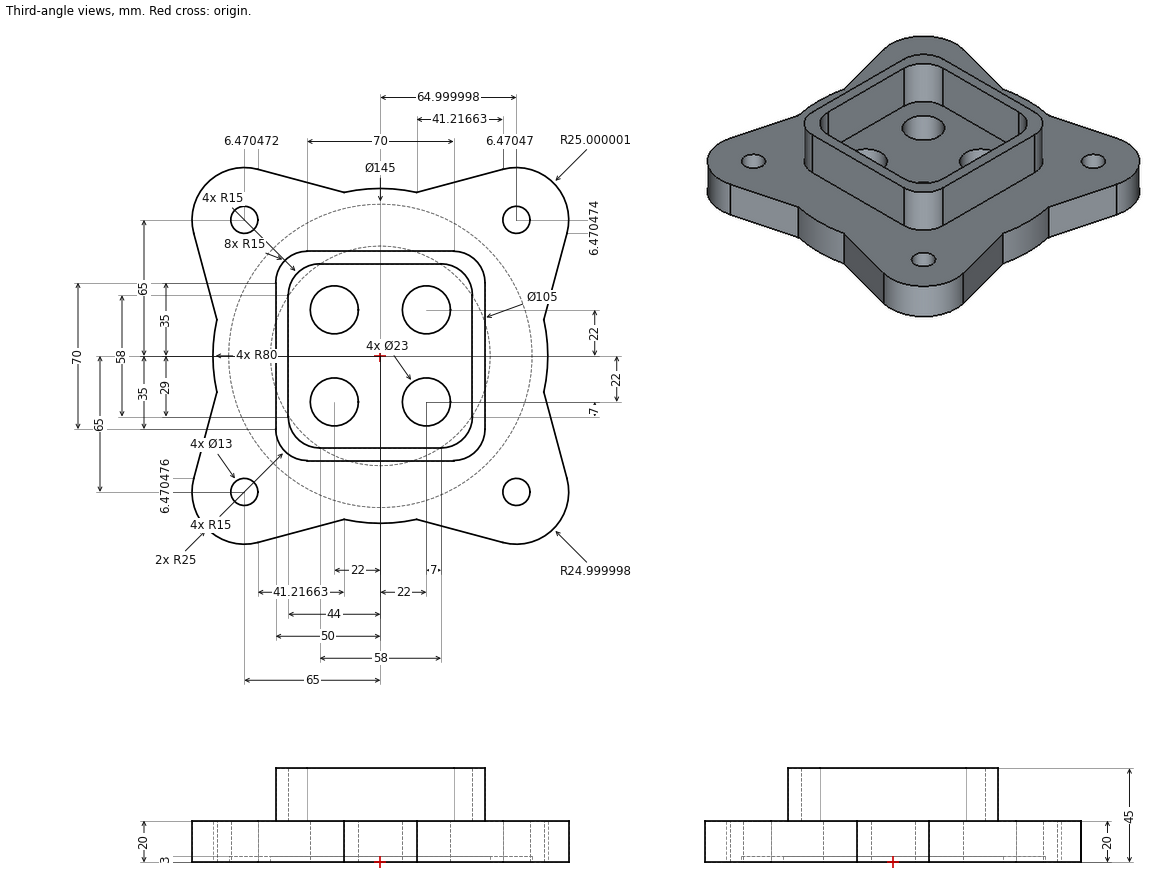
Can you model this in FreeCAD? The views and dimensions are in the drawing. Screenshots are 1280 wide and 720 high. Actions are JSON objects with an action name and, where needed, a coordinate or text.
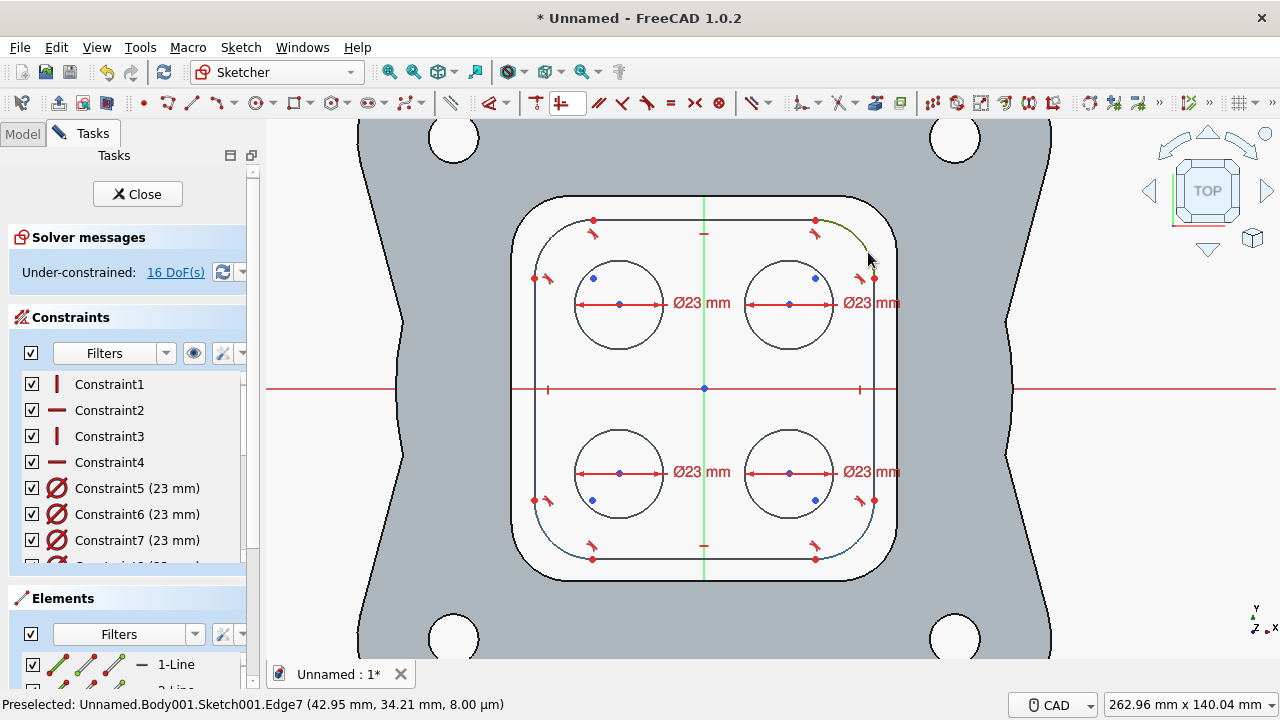
{"action": "left_click", "coordinate": [567, 226]}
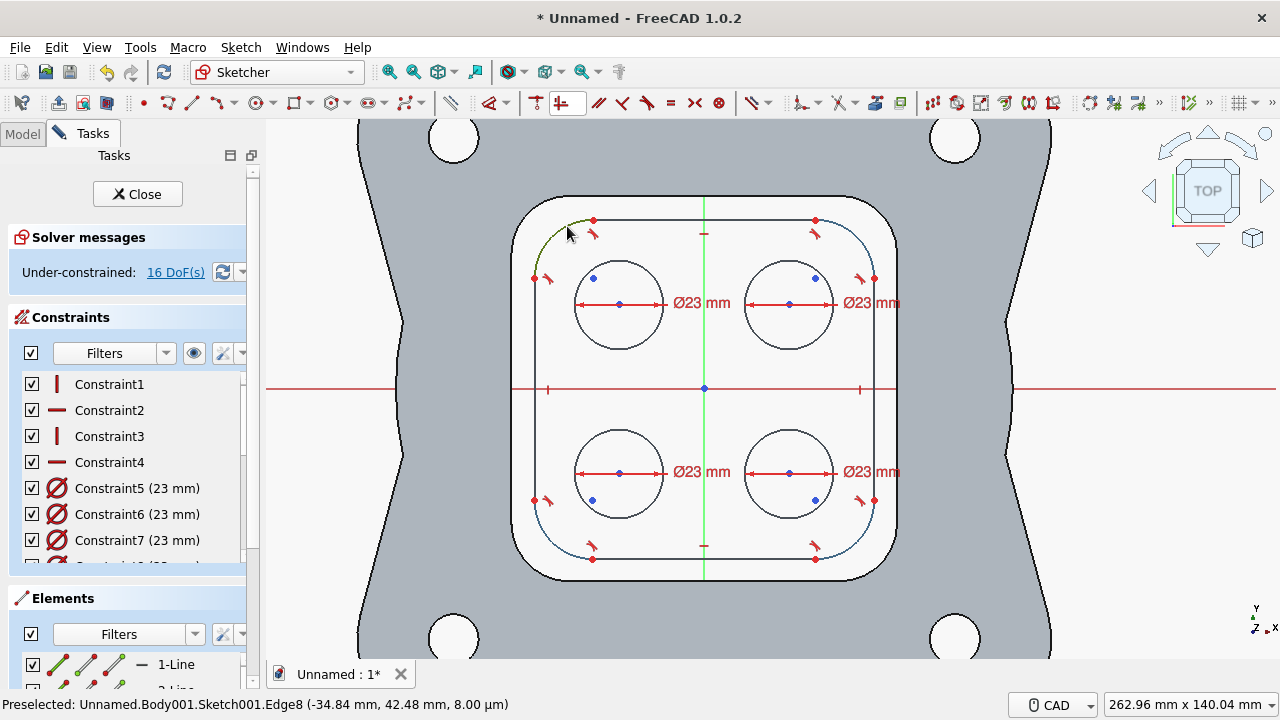
{"action": "left_click", "coordinate": [672, 104]}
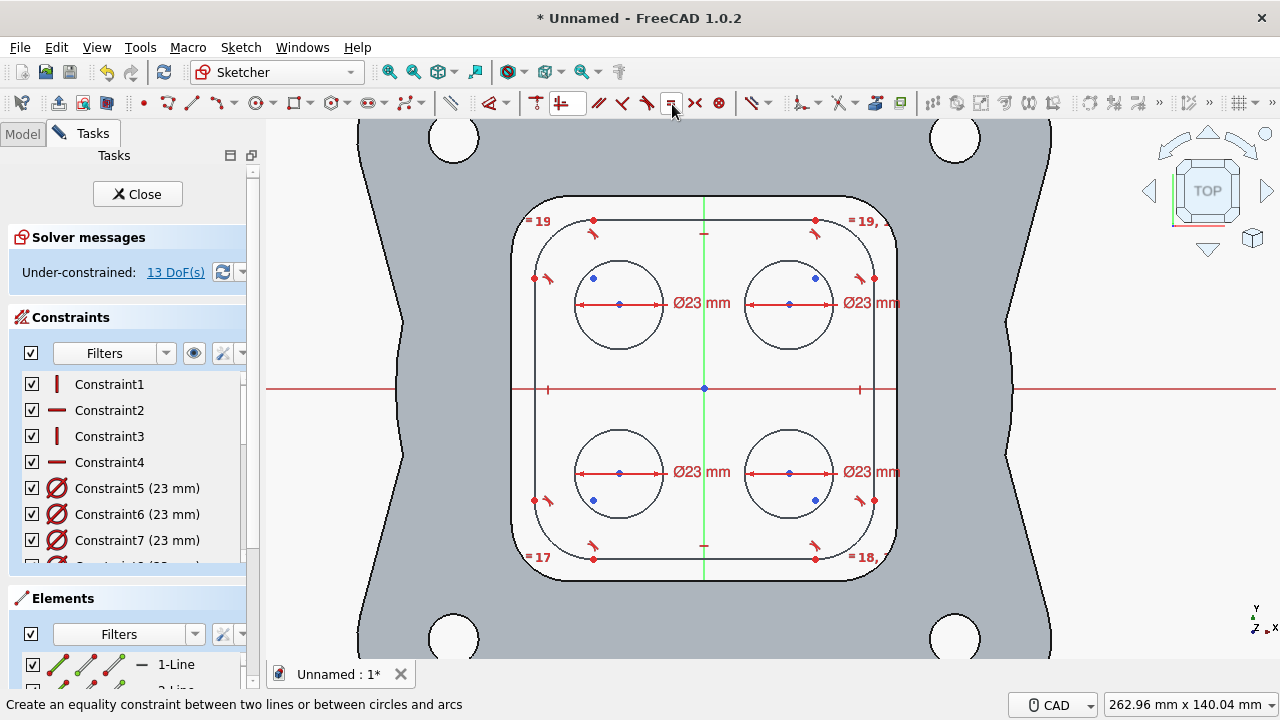
{"action": "left_click", "coordinate": [789, 474]}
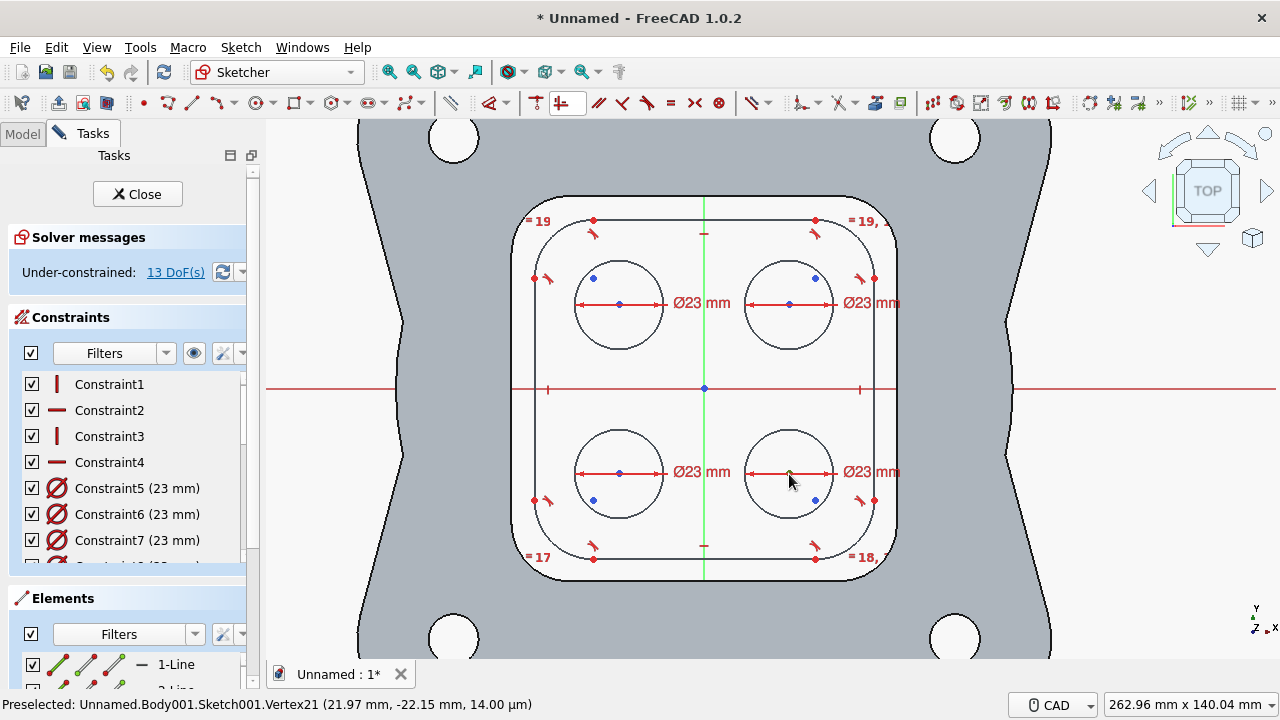
{"action": "left_click", "coordinate": [619, 474]}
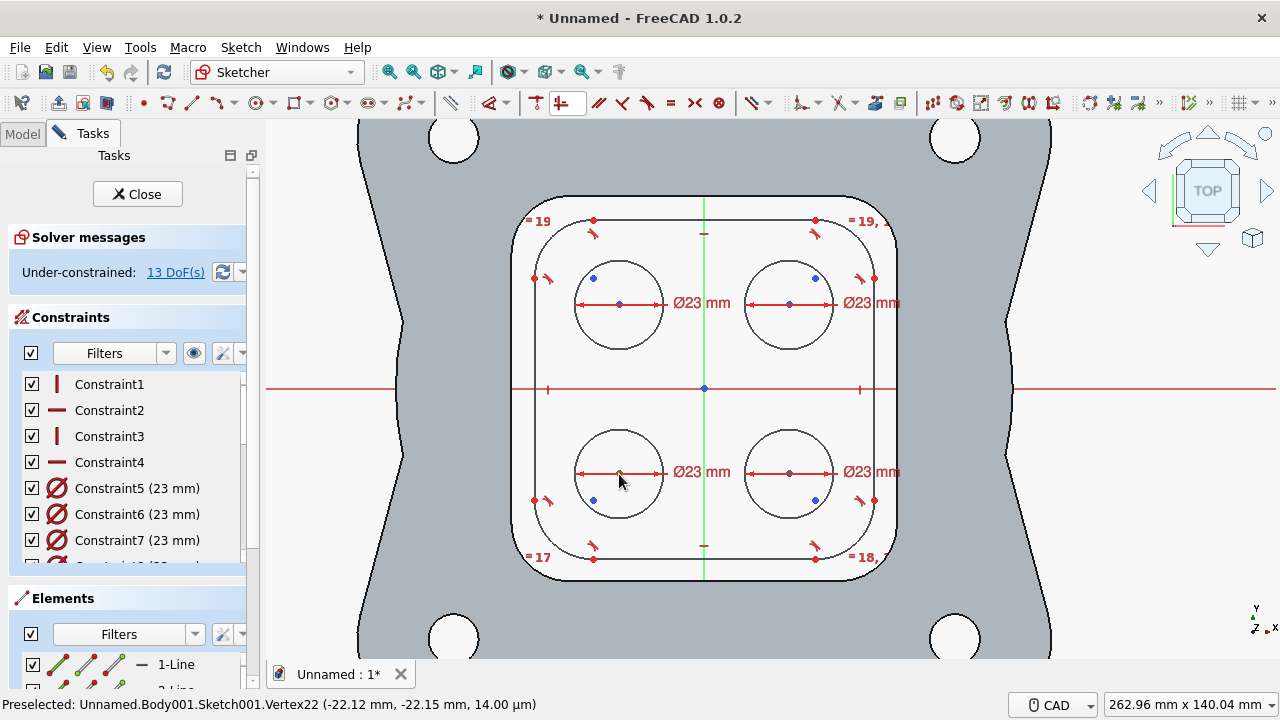
{"action": "key", "text": "h"}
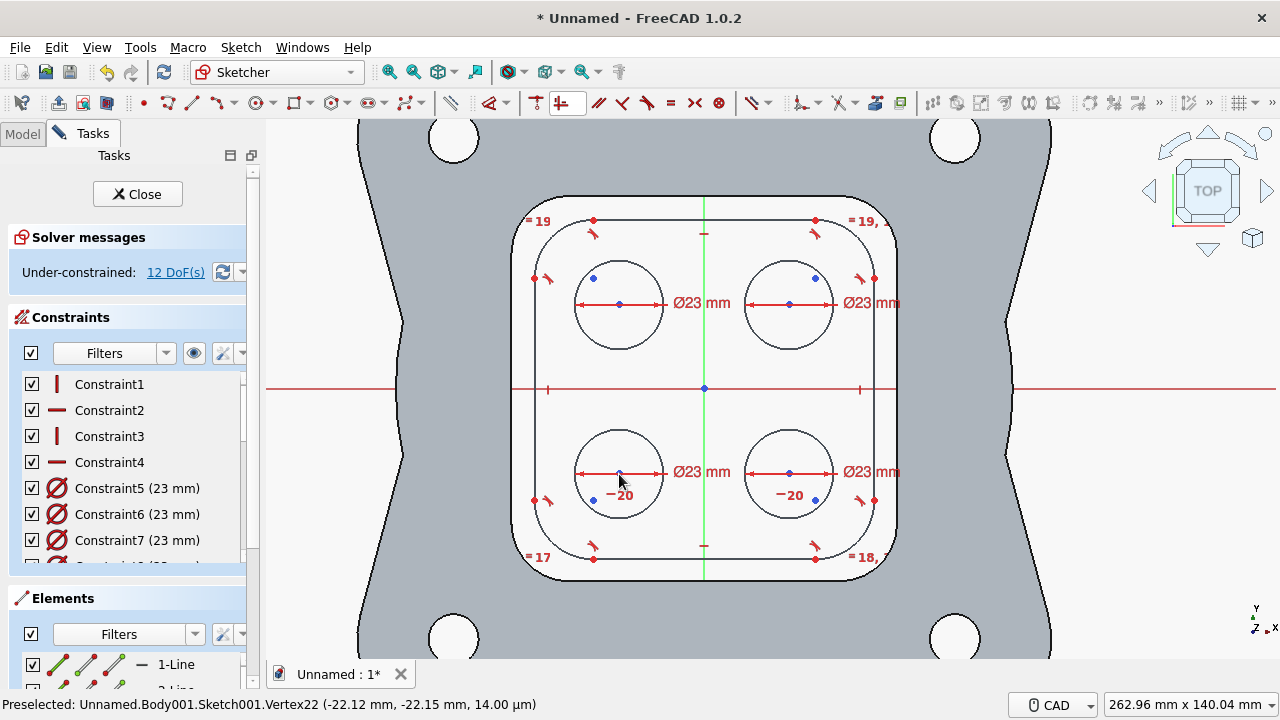
{"action": "left_click", "coordinate": [789, 474]}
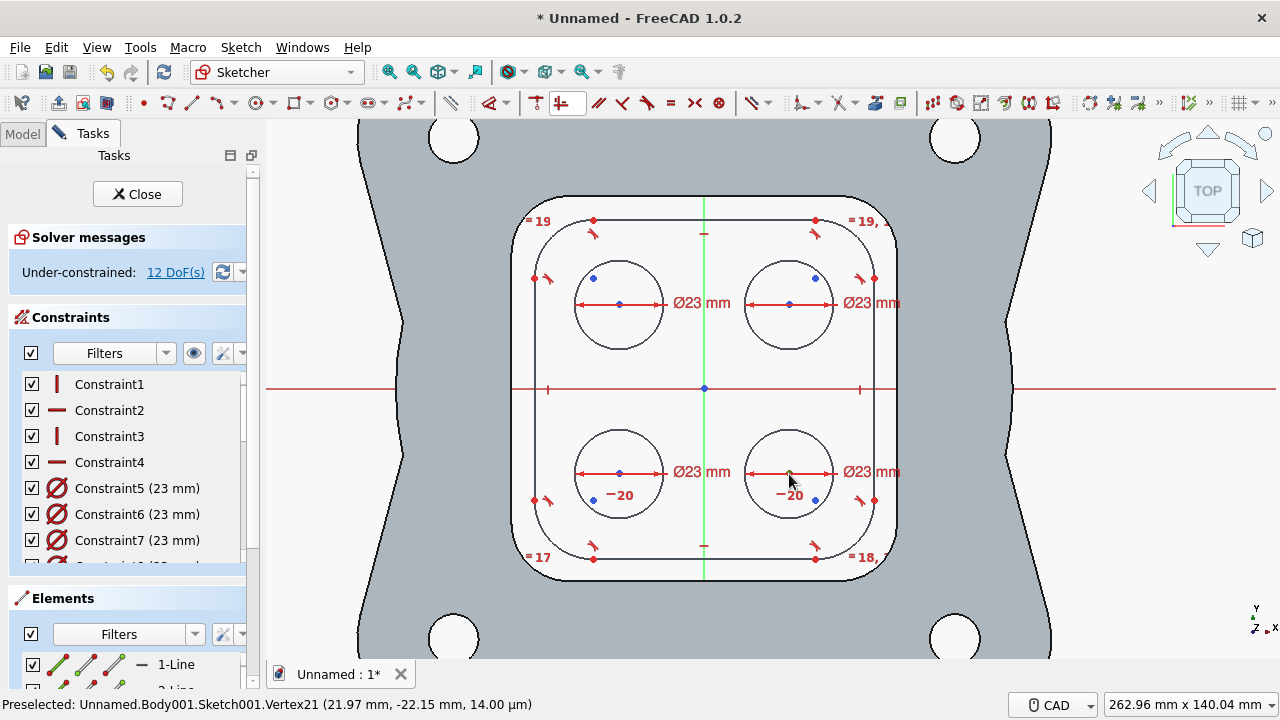
{"action": "left_click", "coordinate": [789, 305]}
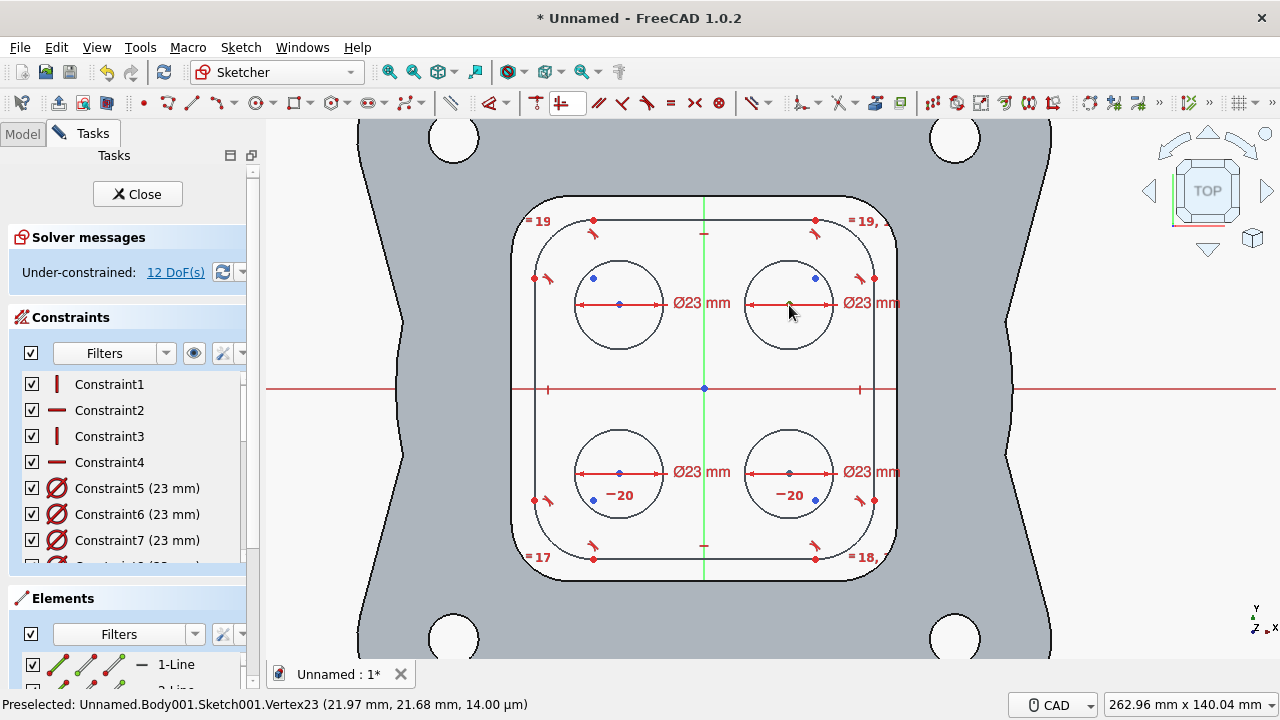
{"action": "key", "text": "v"}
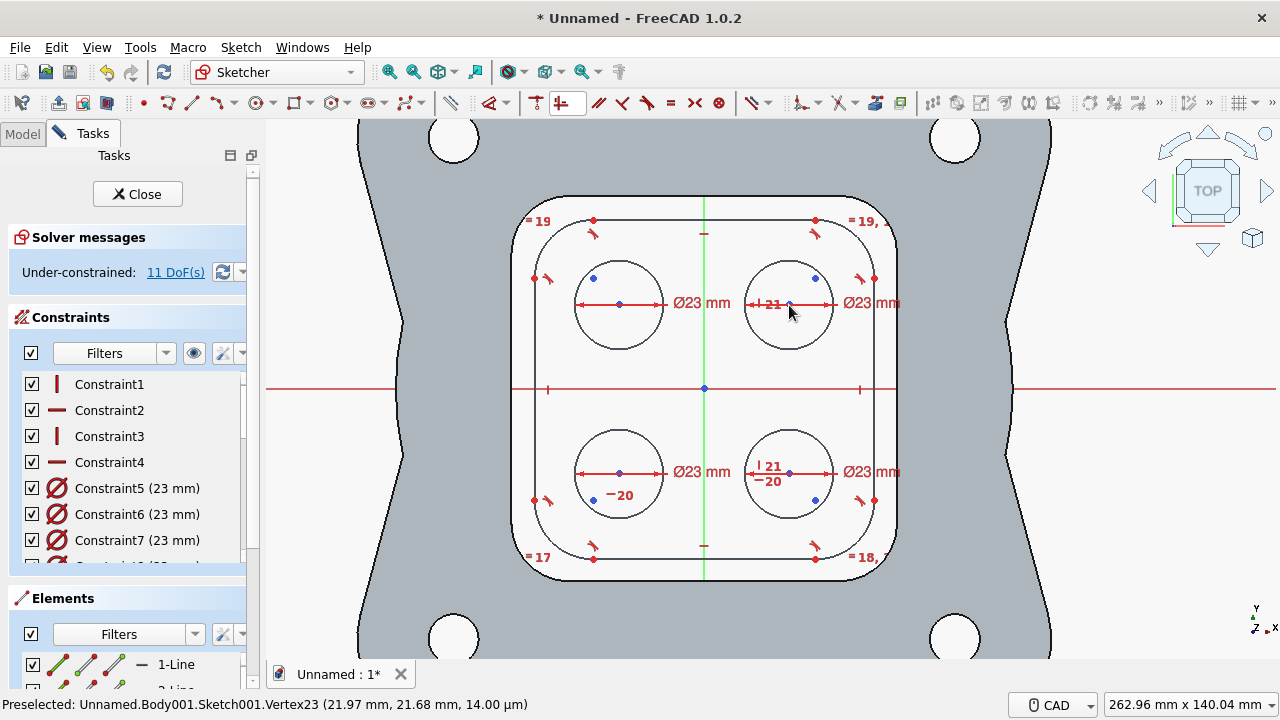
{"action": "left_click", "coordinate": [619, 474]}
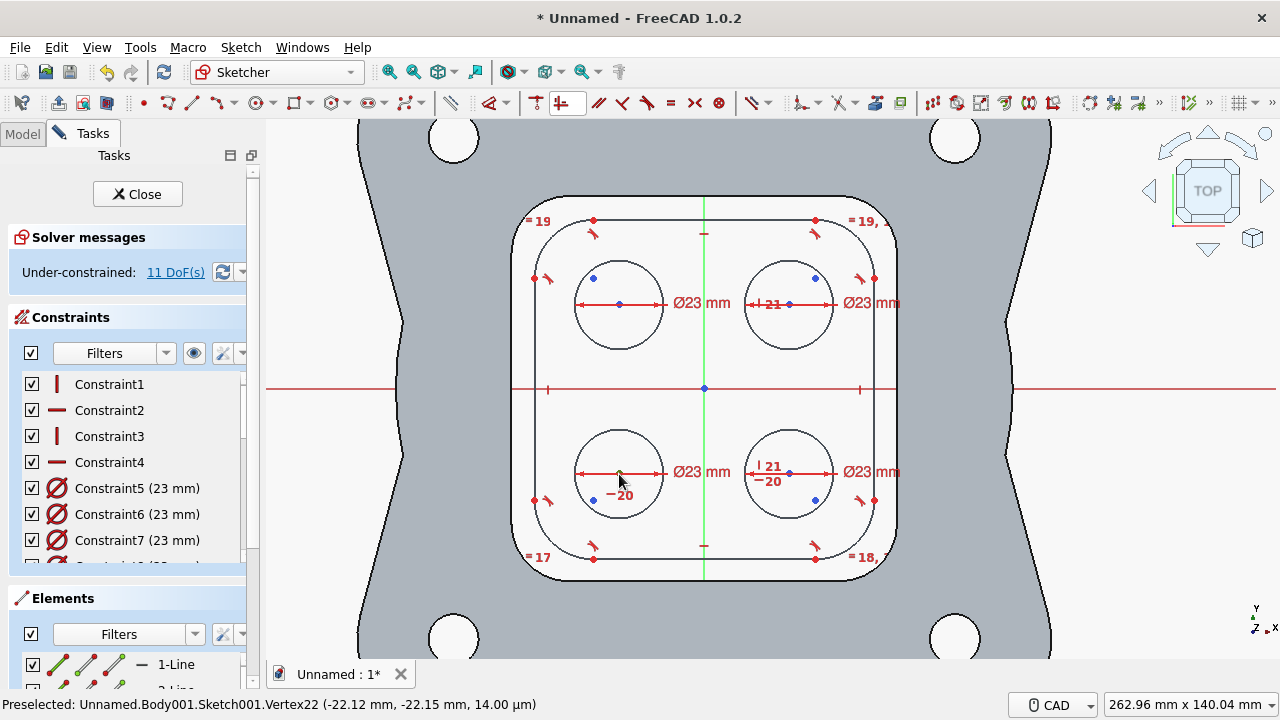
{"action": "left_click", "coordinate": [619, 305]}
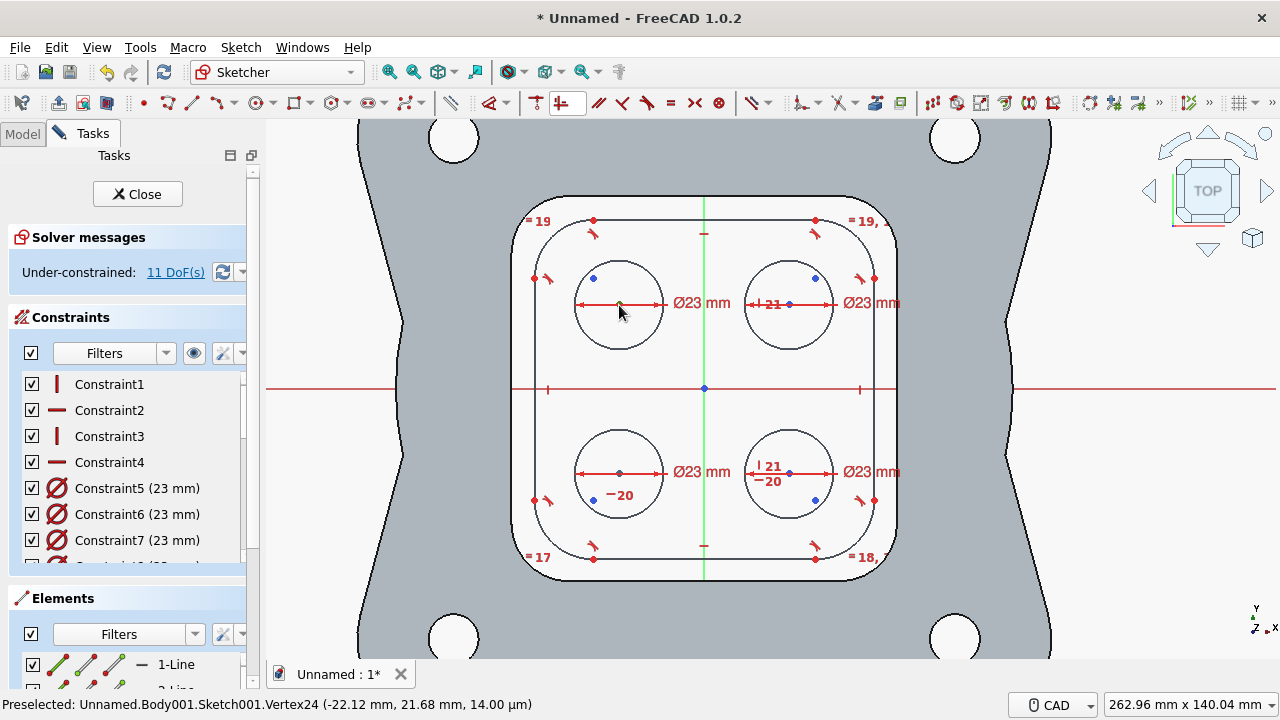
{"action": "left_click", "coordinate": [580, 104]}